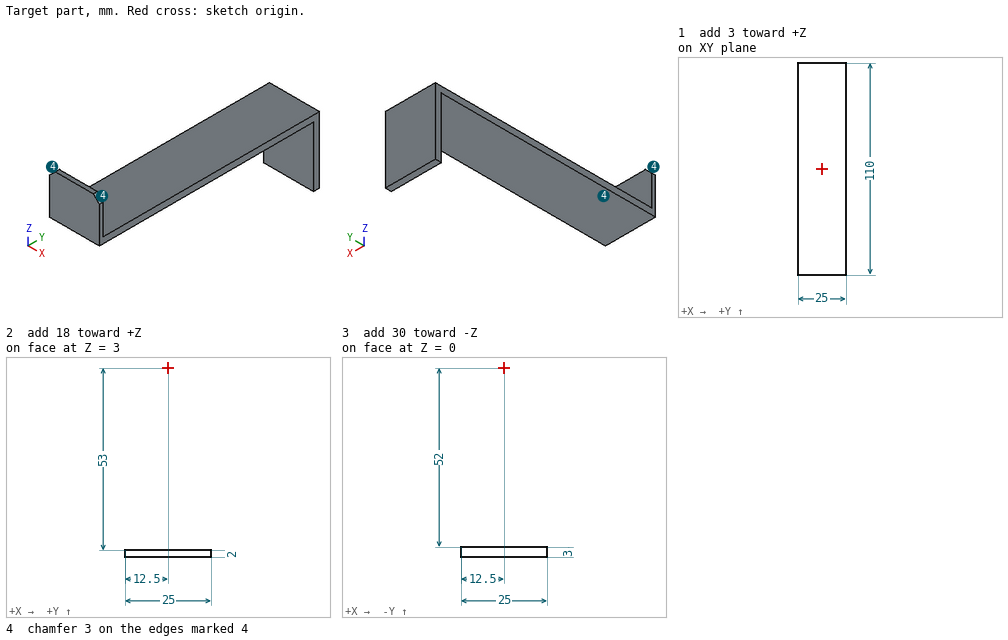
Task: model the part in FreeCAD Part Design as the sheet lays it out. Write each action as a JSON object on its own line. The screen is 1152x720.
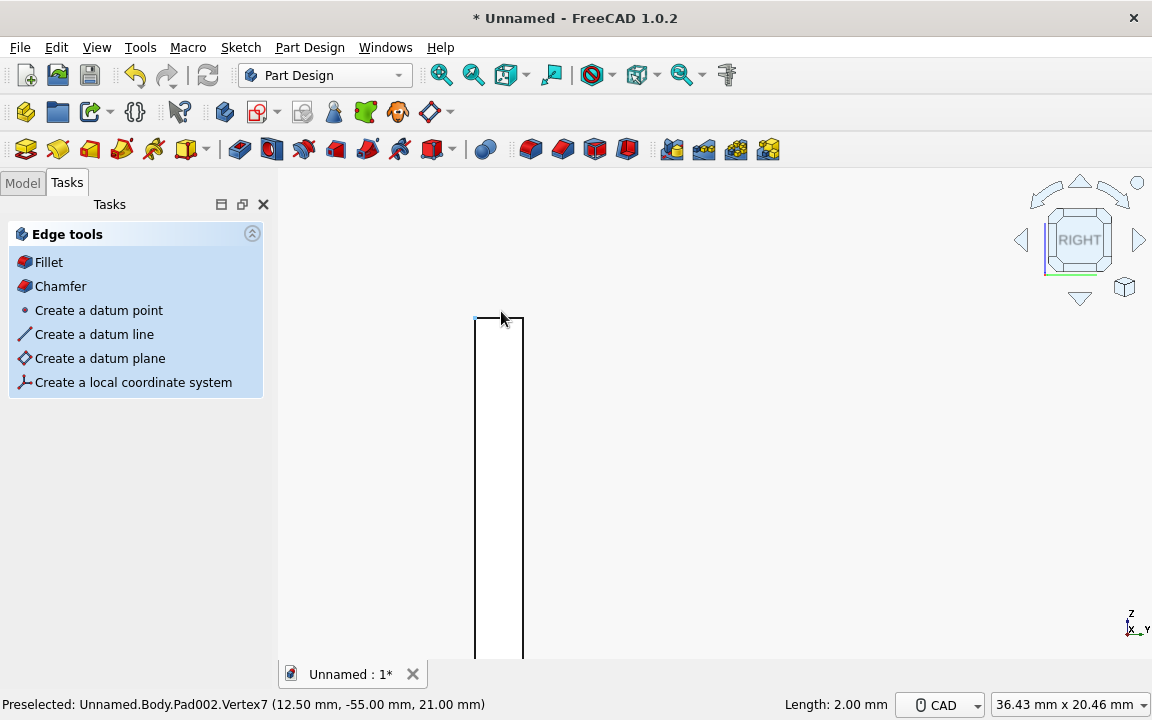
{"action": "left_click", "coordinate": [499, 317], "text": "ctrl"}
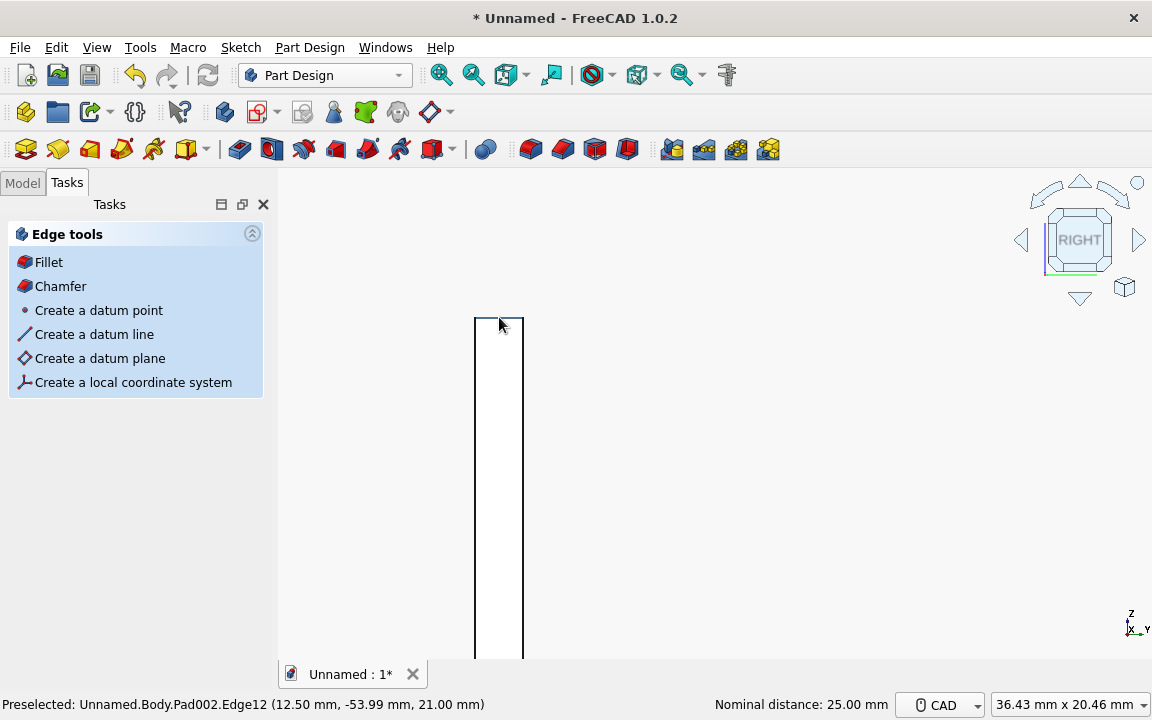
{"action": "left_click", "coordinate": [564, 150]}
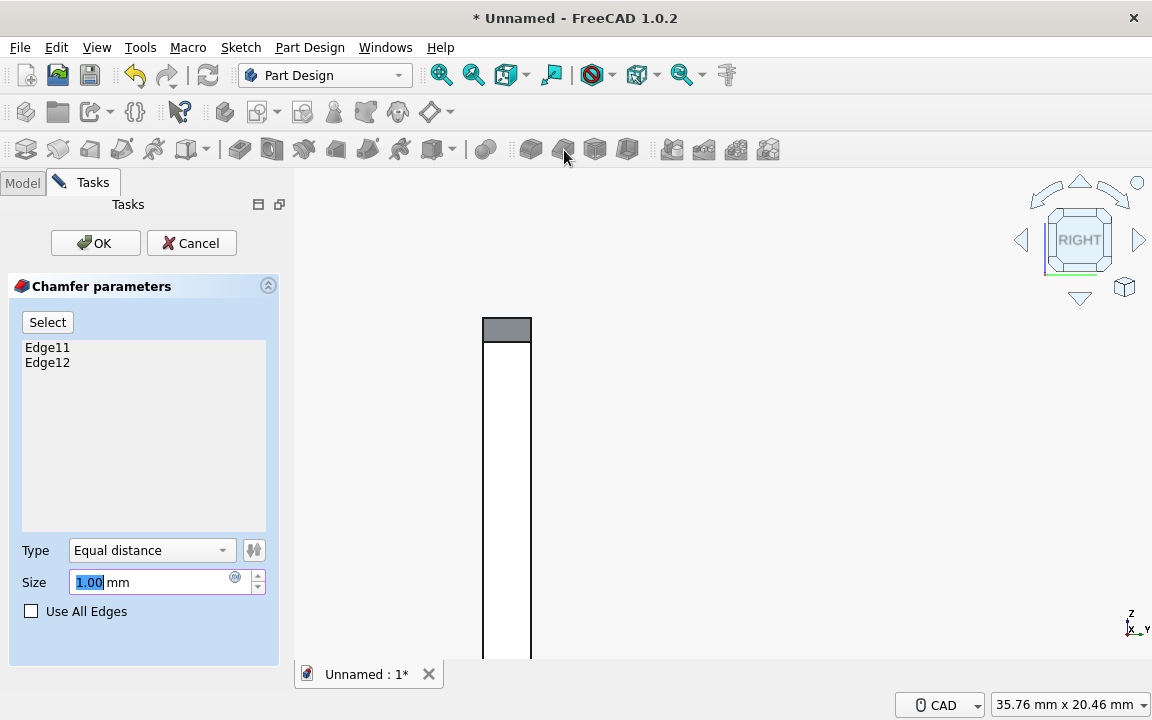
{"action": "type", "text": "3"}
{"action": "key", "text": "Tab"}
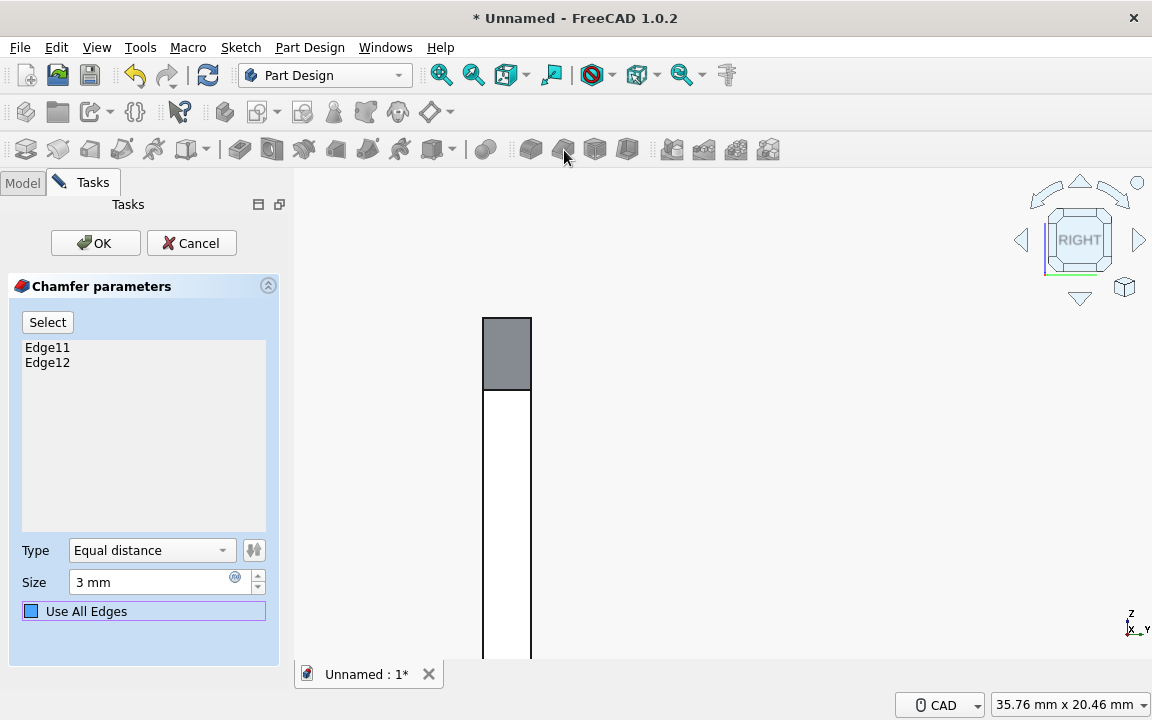
{"action": "left_click", "coordinate": [96, 243]}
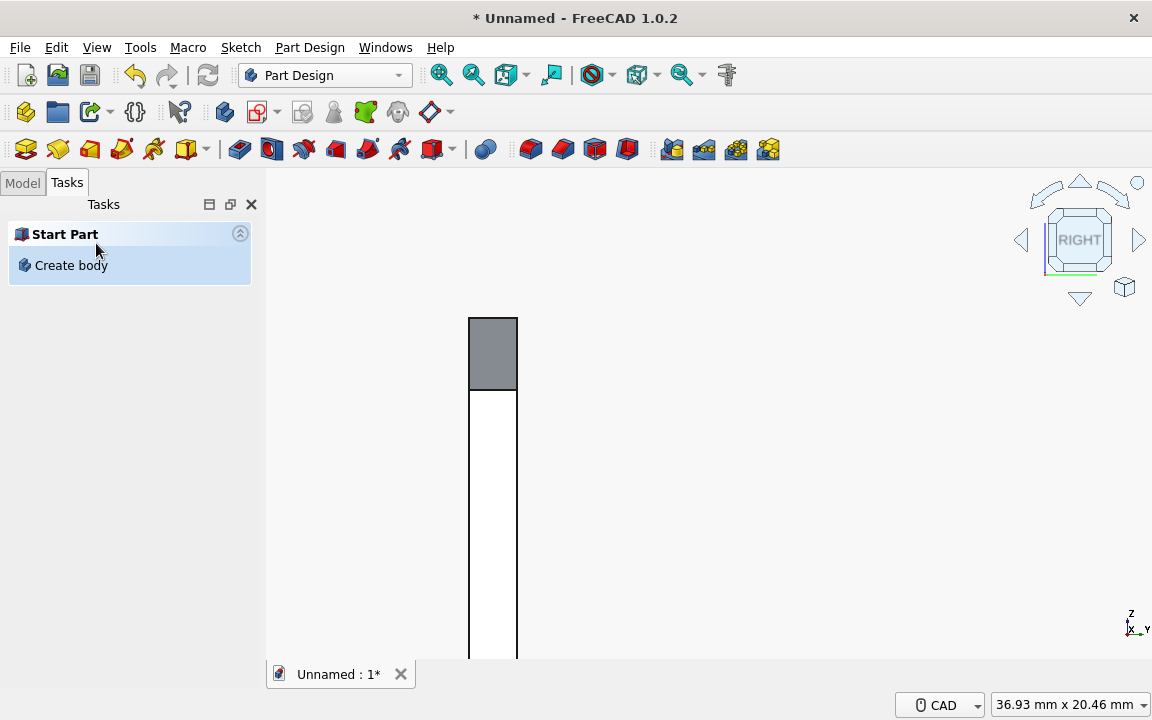
{"action": "key", "text": "0"}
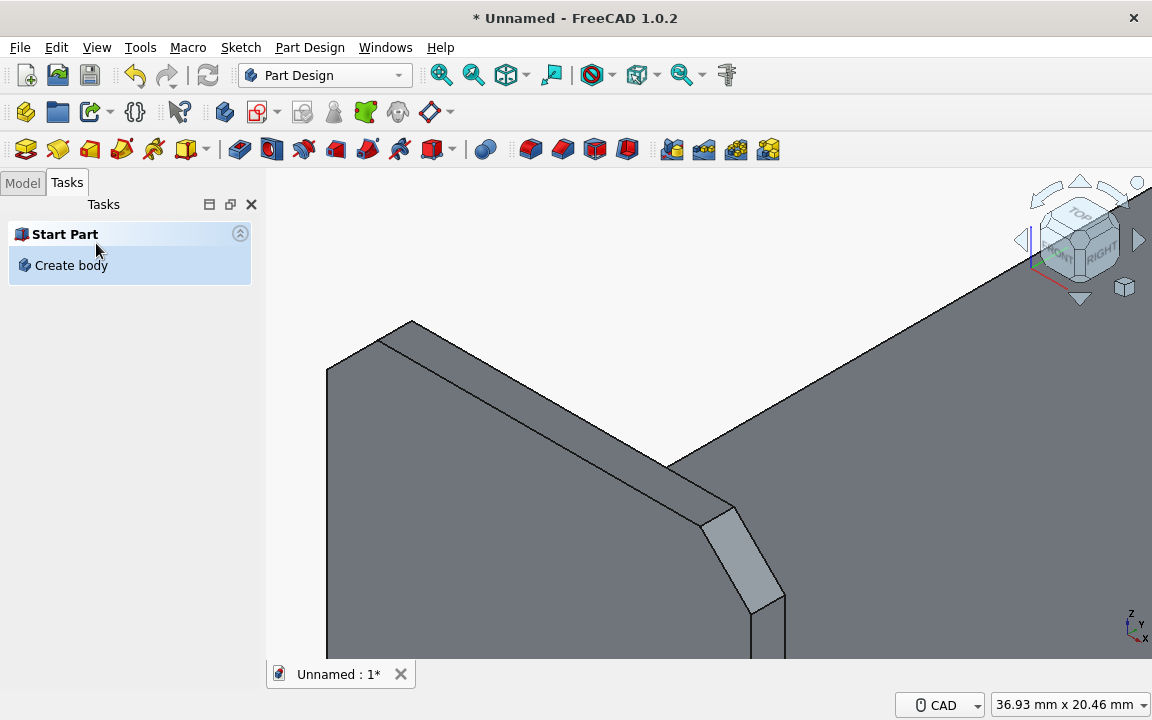
{"action": "key", "text": "v f"}